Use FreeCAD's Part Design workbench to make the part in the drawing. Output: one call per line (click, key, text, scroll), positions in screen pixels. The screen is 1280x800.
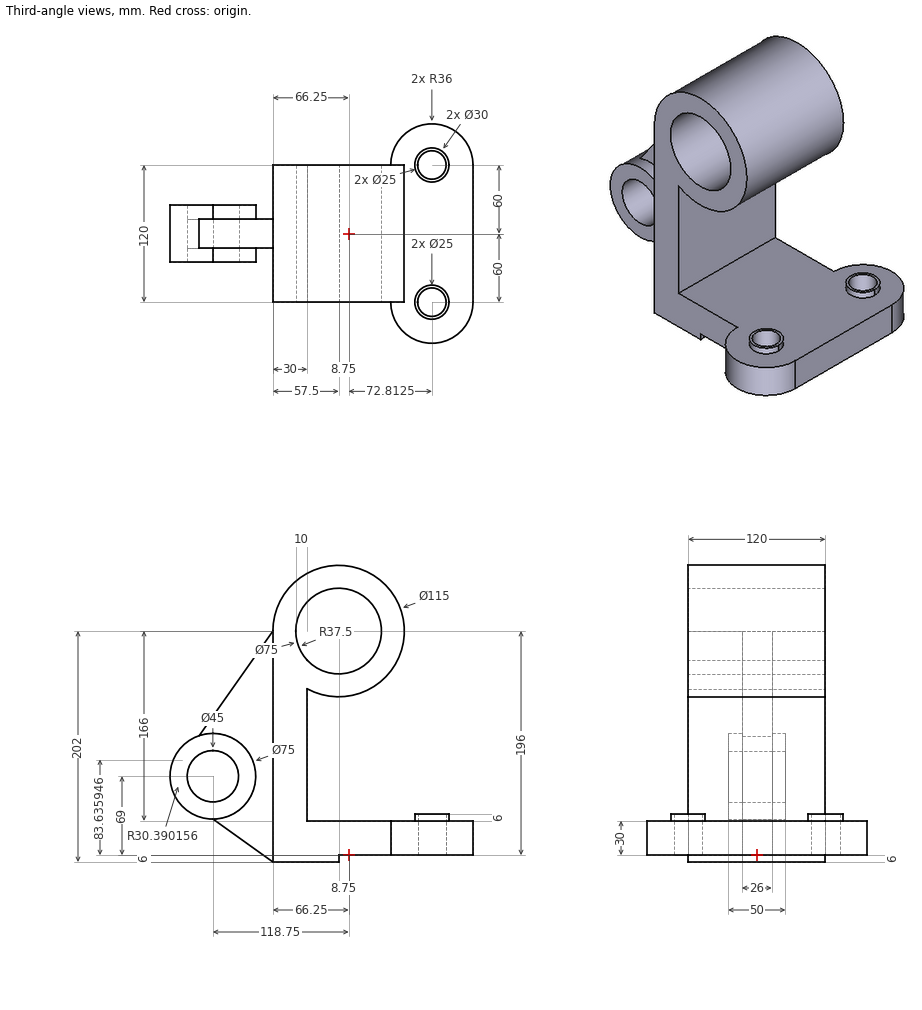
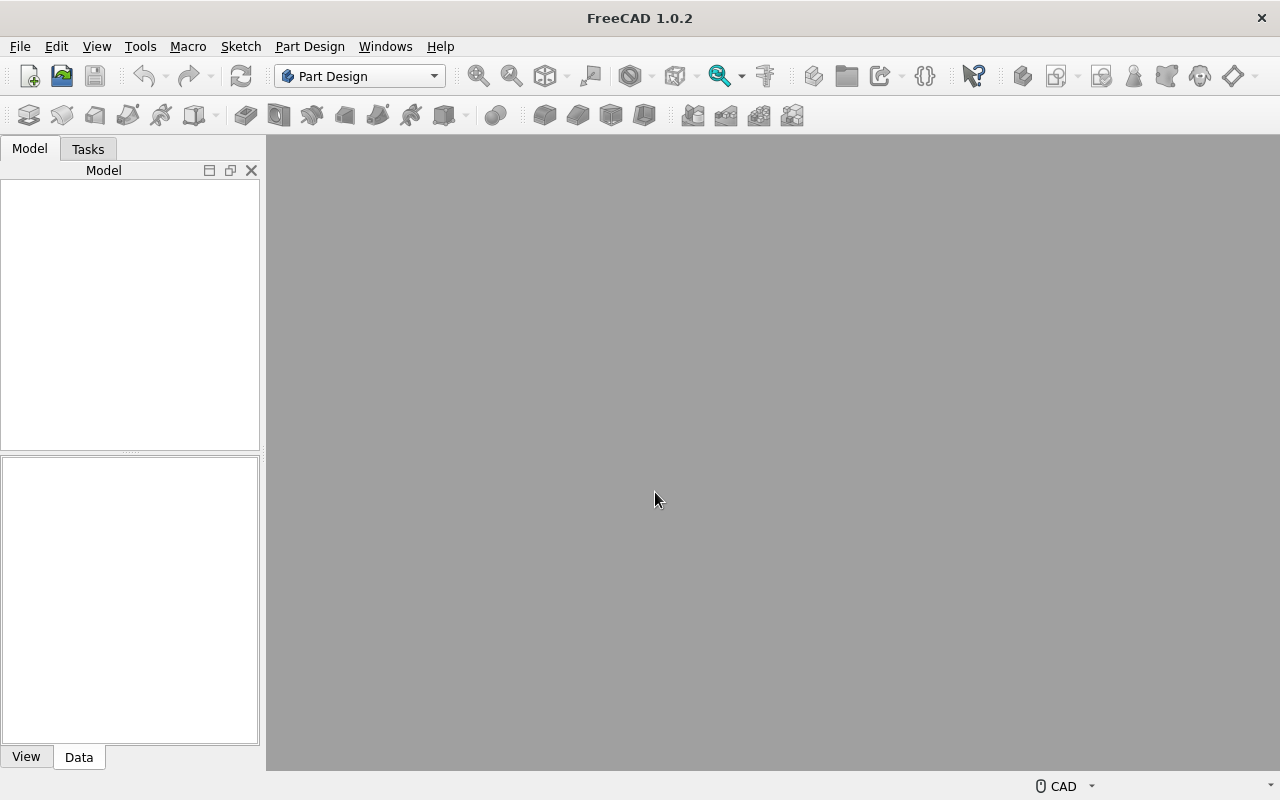
key(ctrl+n)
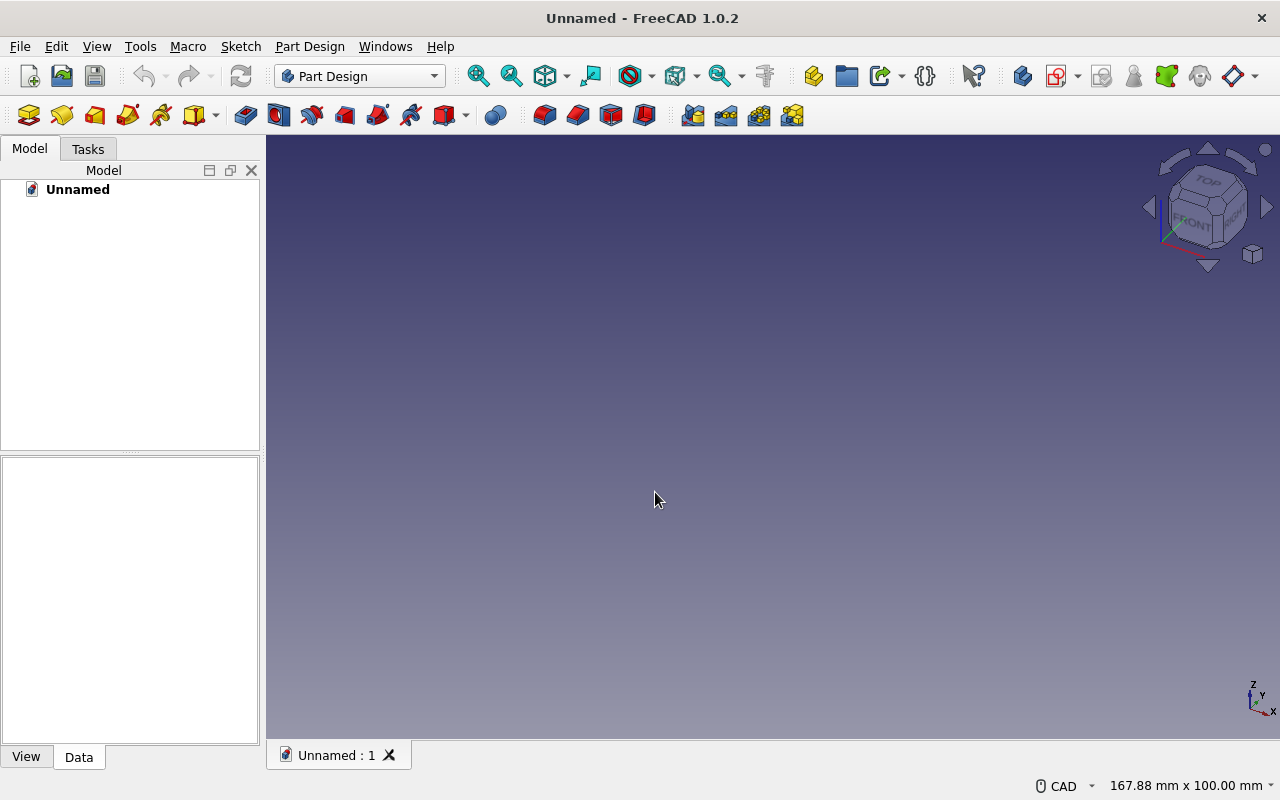
click(1056, 76)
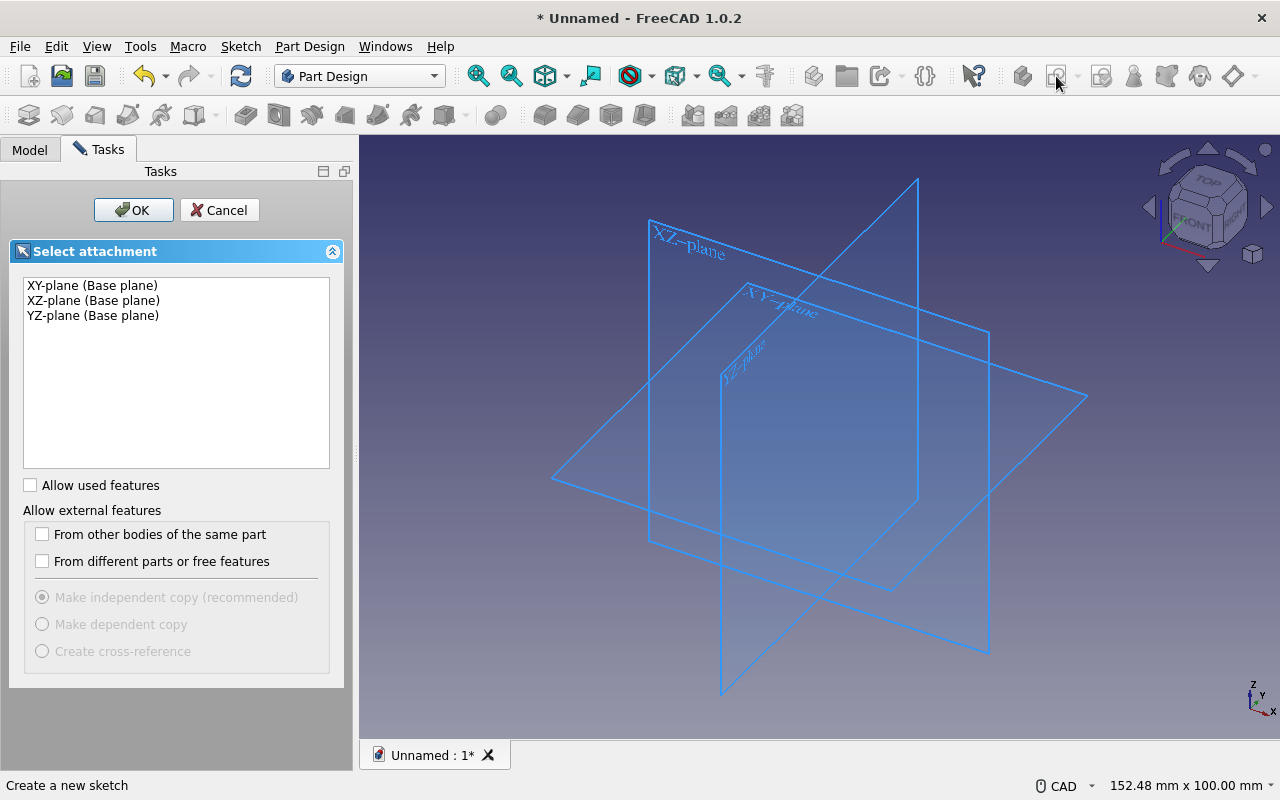
click(84, 286)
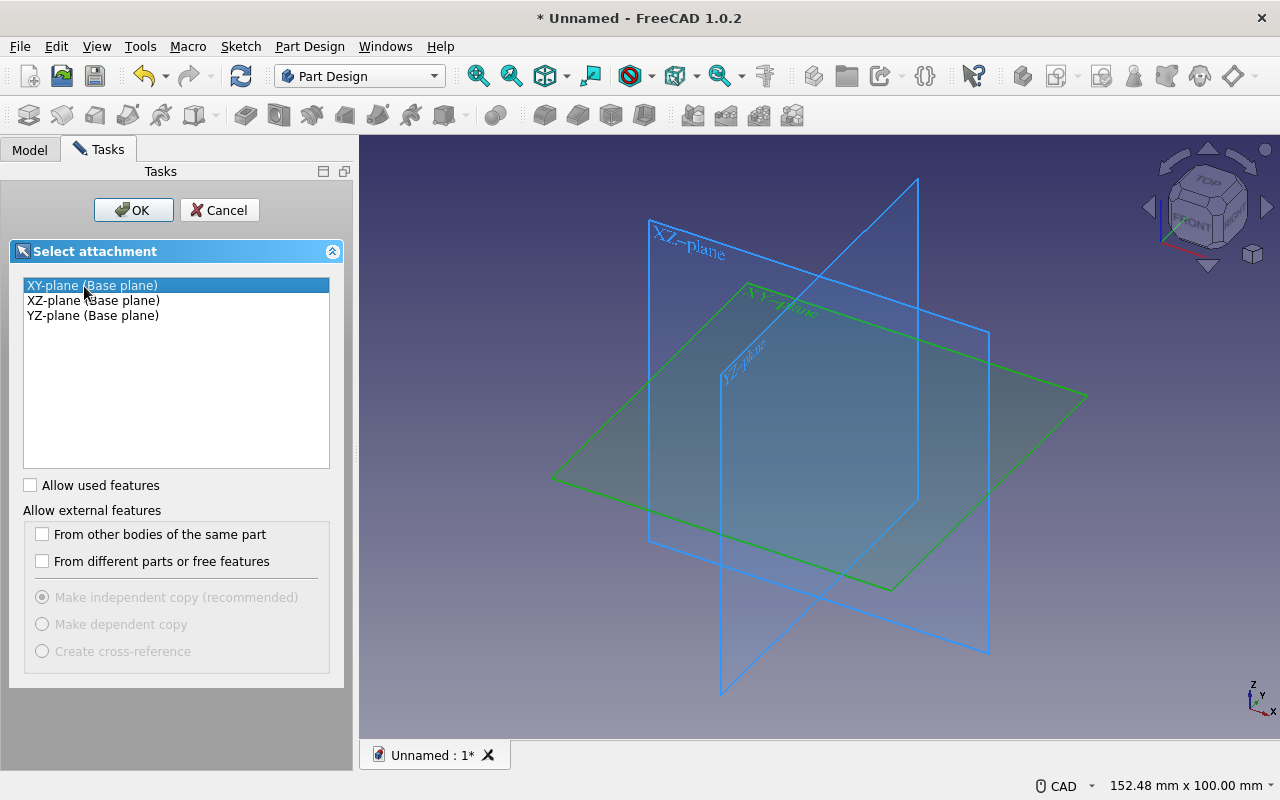
click(134, 210)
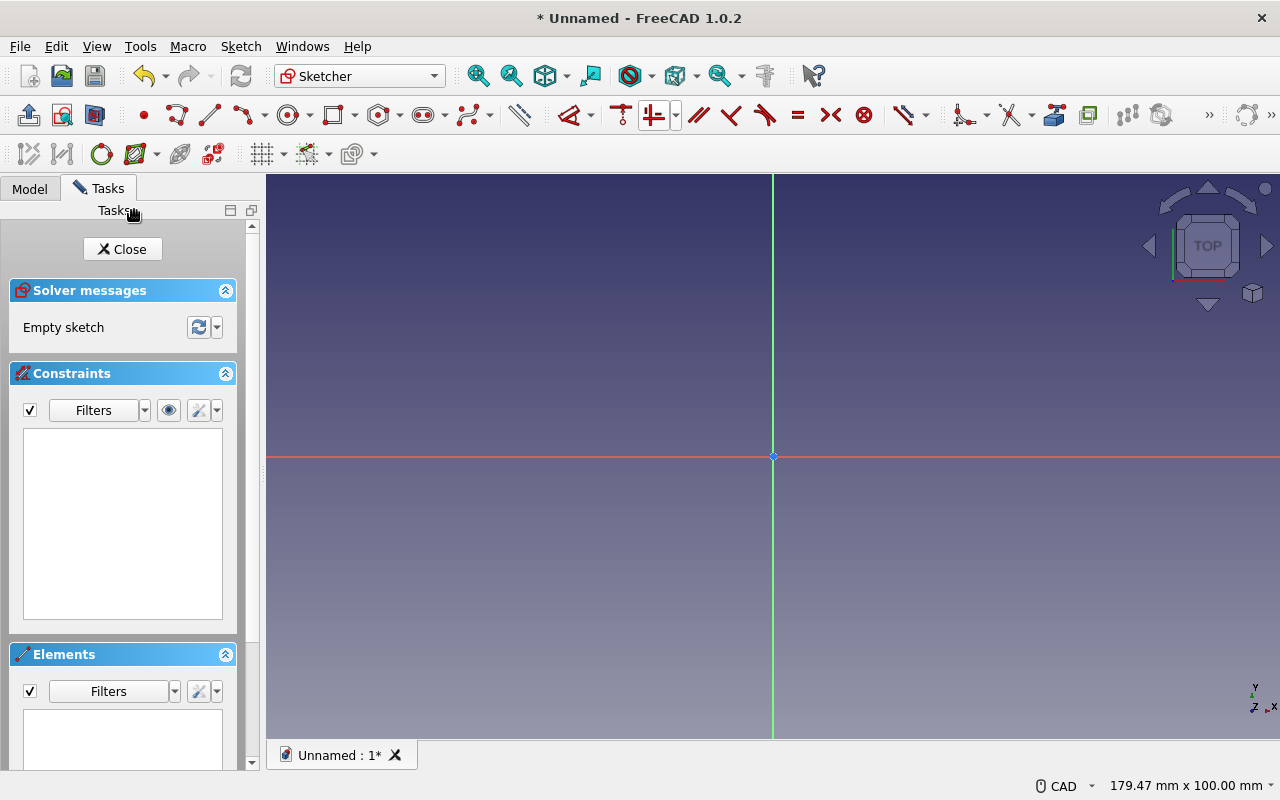
scroll(623, 456, down, 6)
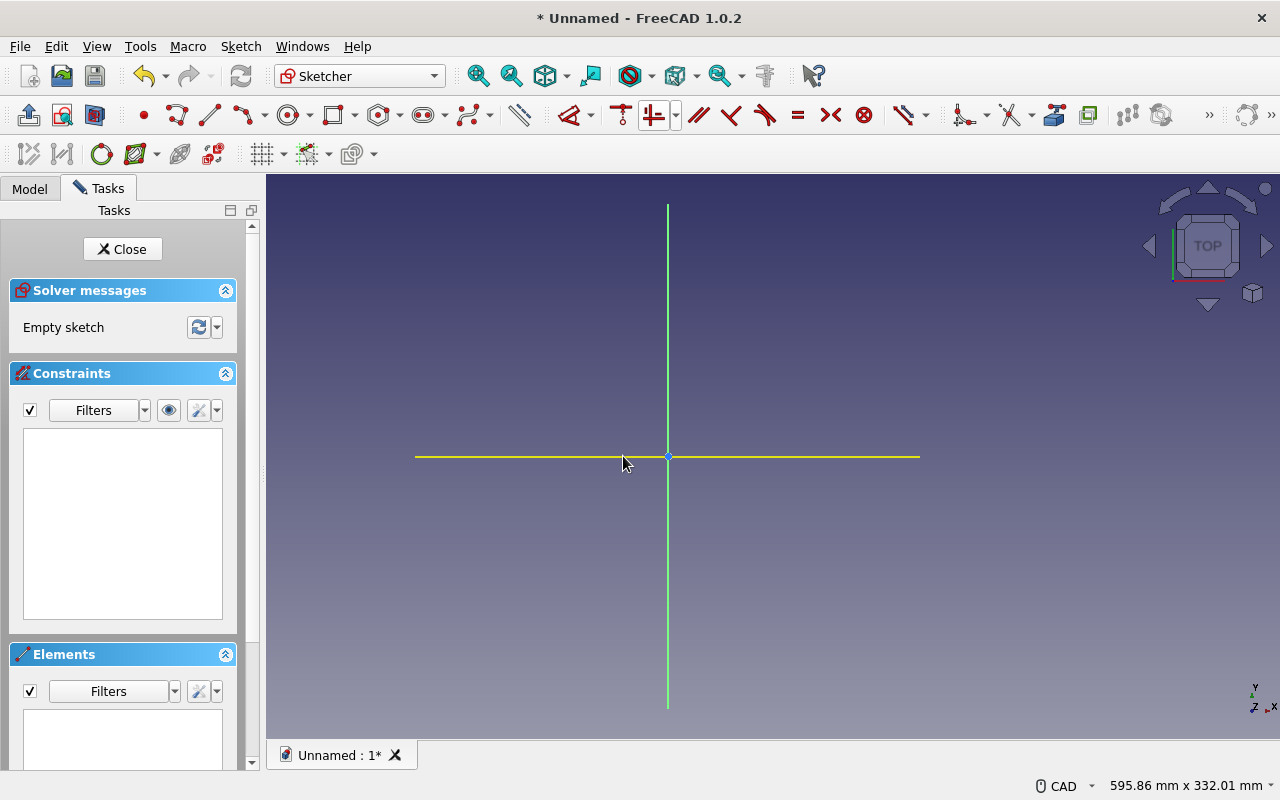
click(210, 116)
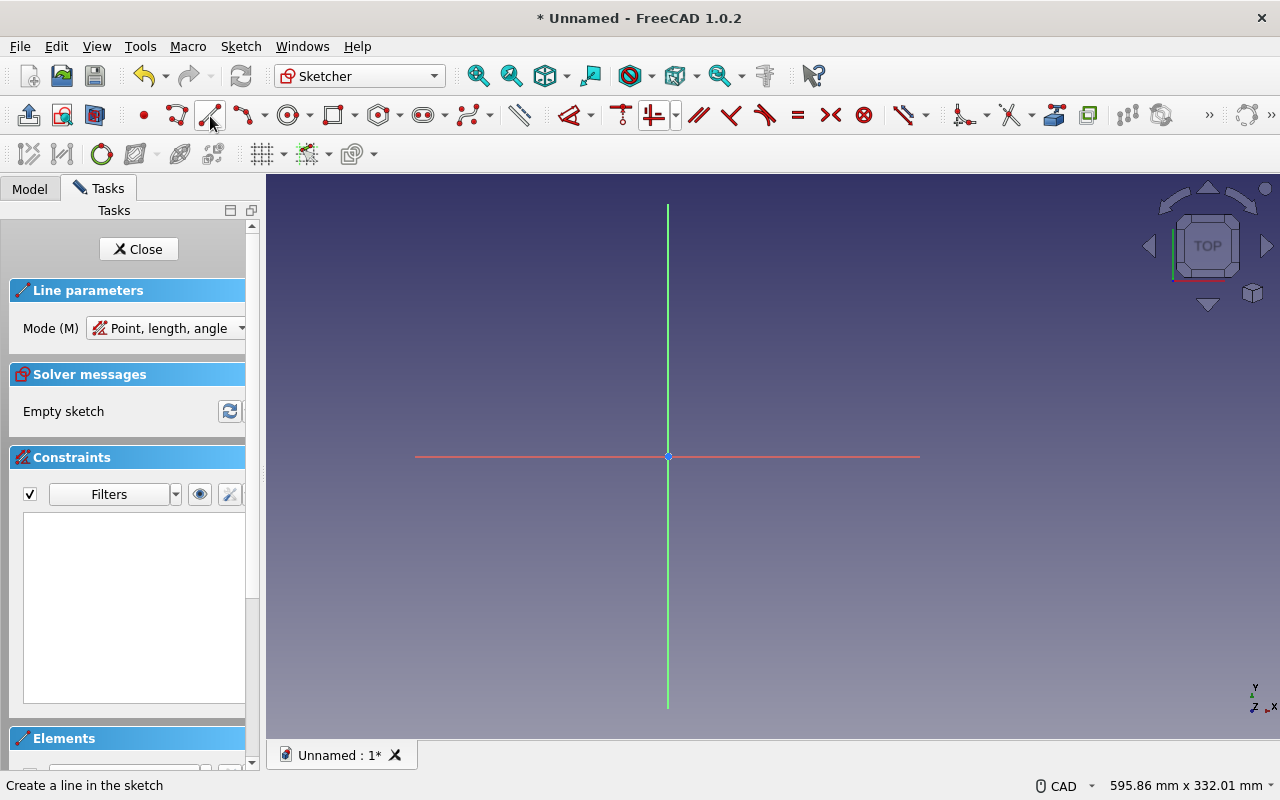
click(854, 559)
click(854, 354)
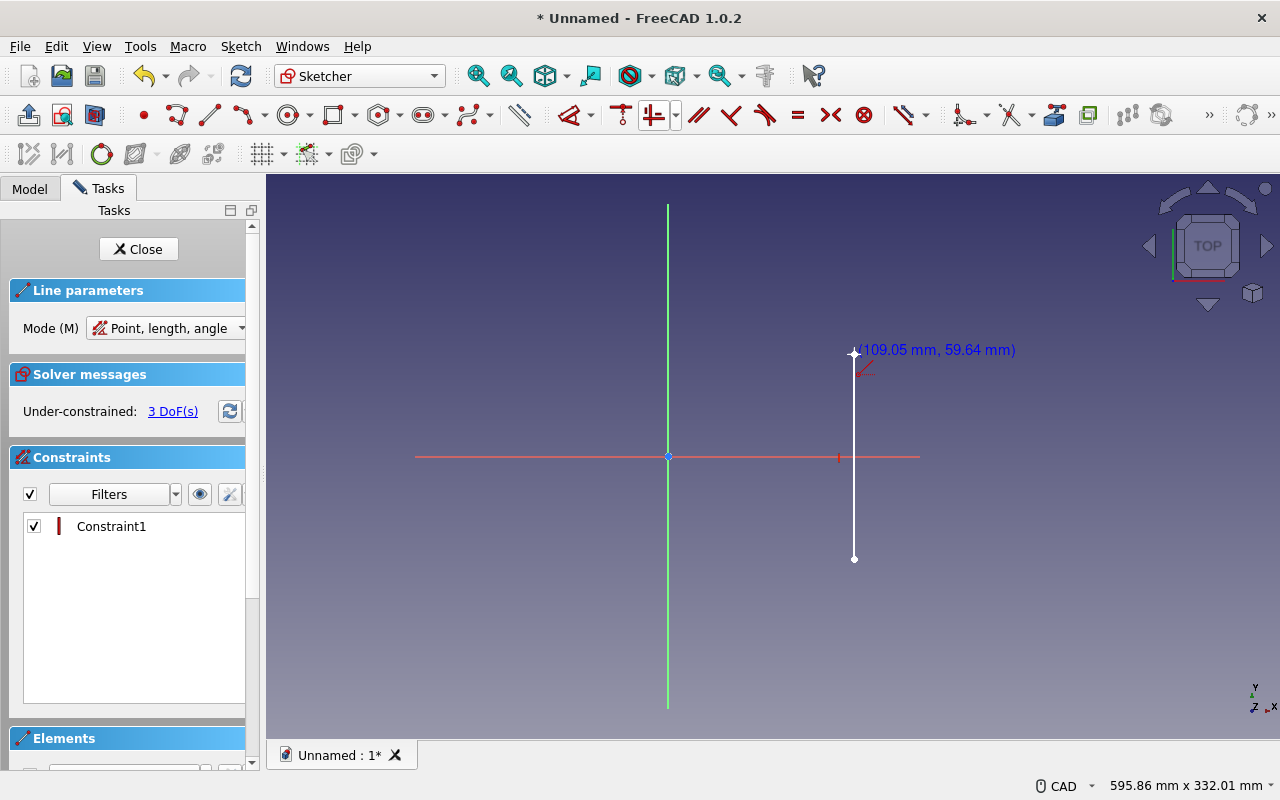
key(g)
key(m)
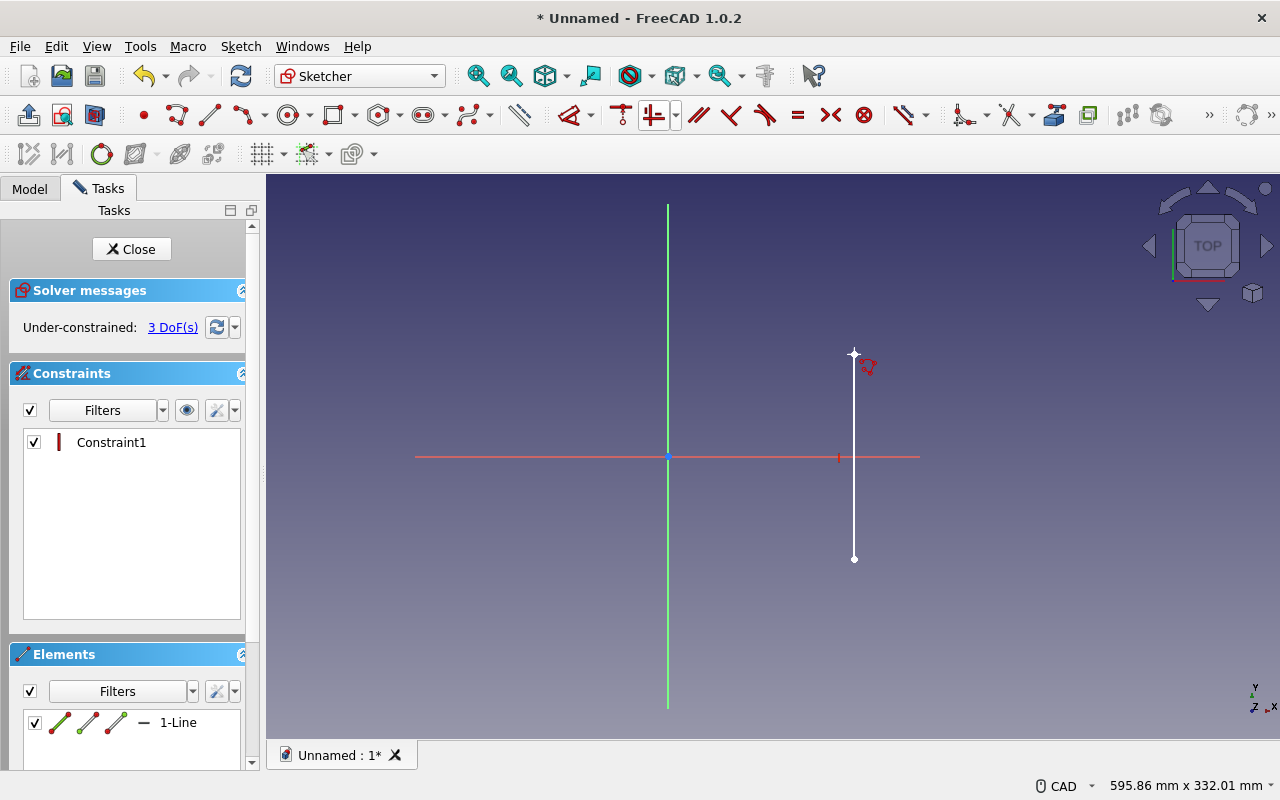
click(731, 354)
click(556, 354)
click(556, 559)
click(731, 559)
right_click(731, 559)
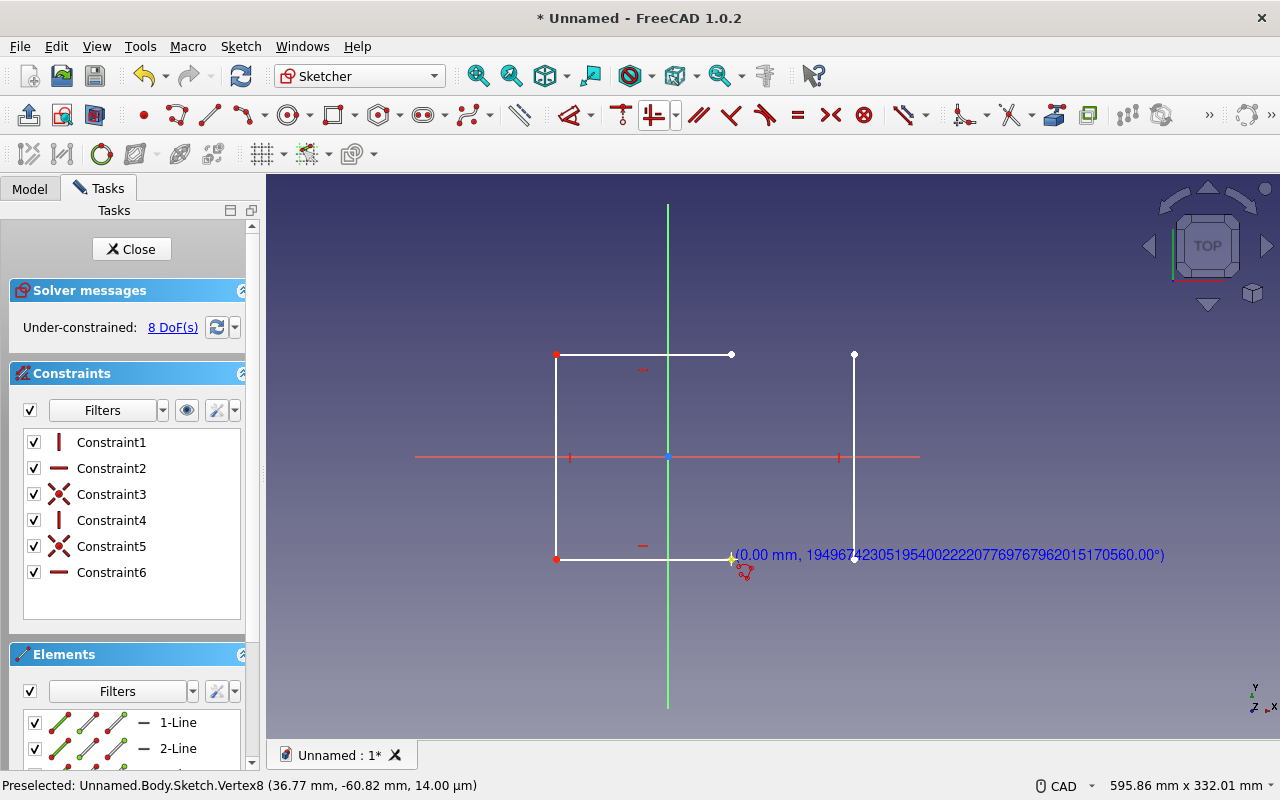
click(242, 116)